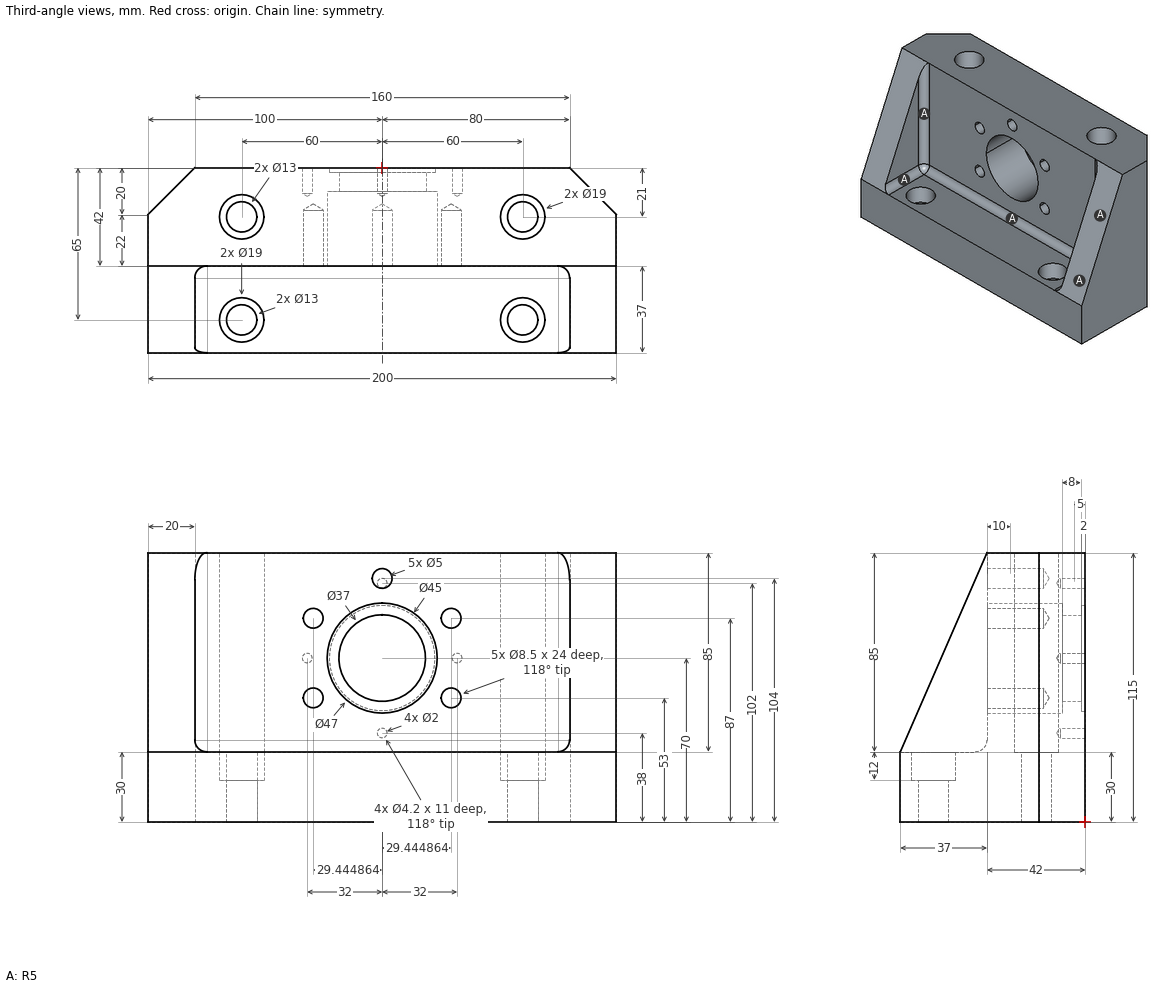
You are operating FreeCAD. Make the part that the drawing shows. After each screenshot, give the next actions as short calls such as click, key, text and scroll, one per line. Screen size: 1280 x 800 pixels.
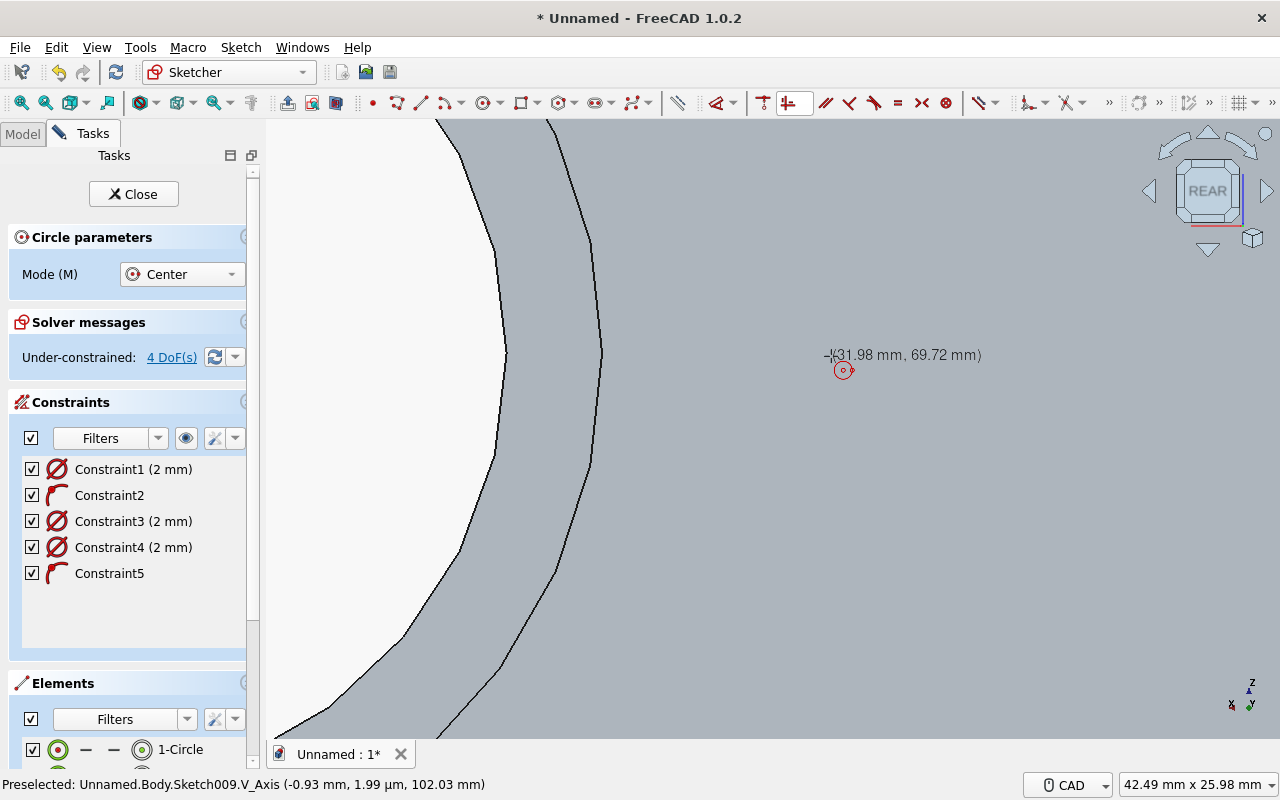
scroll(831, 357, down, 9)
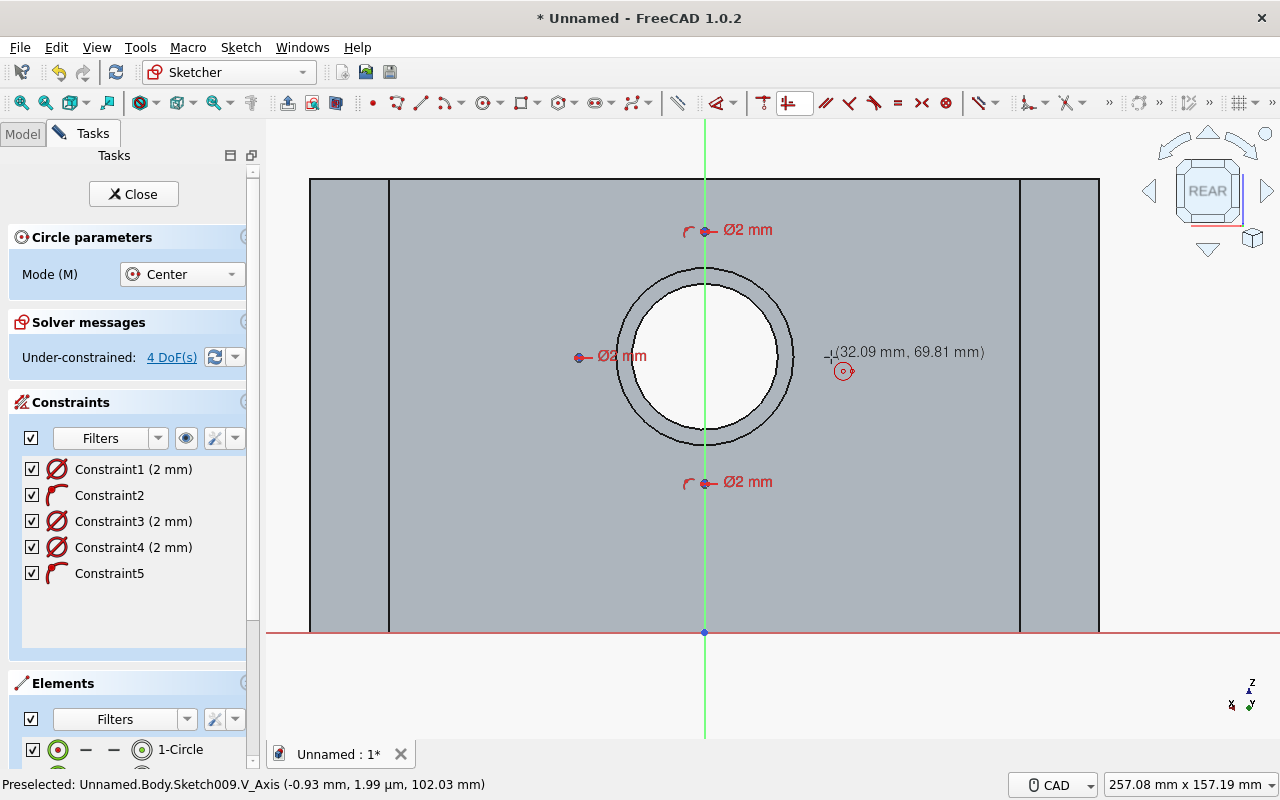
click(831, 357)
move(834, 354)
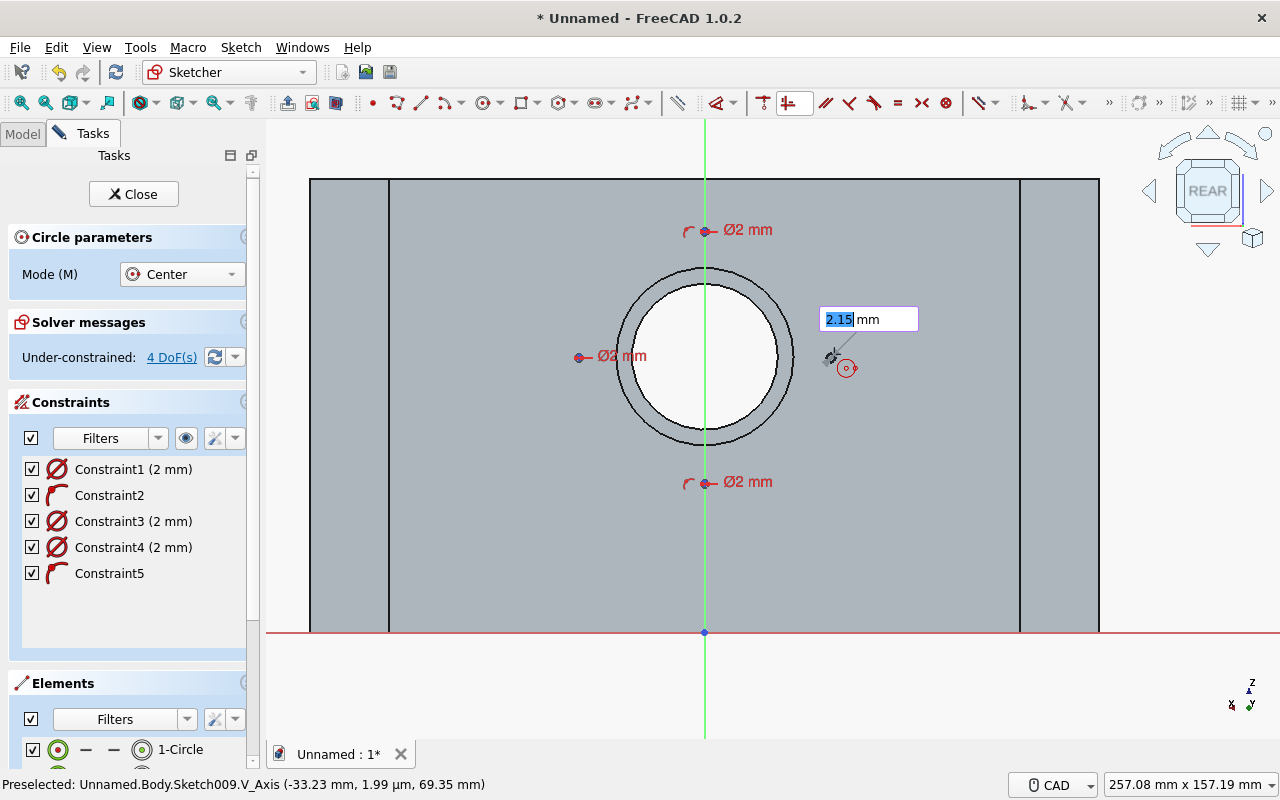
text(2)
key(Return)
key(Escape)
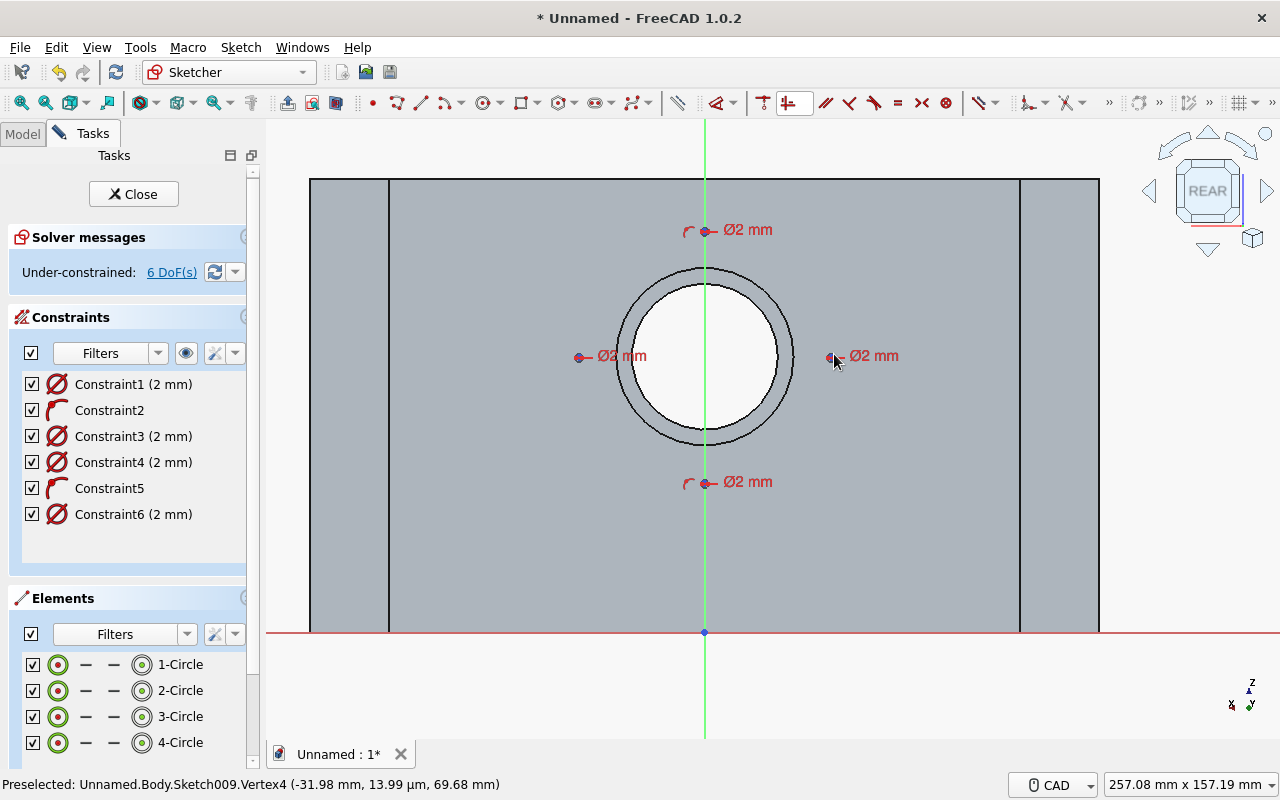
click(579, 358)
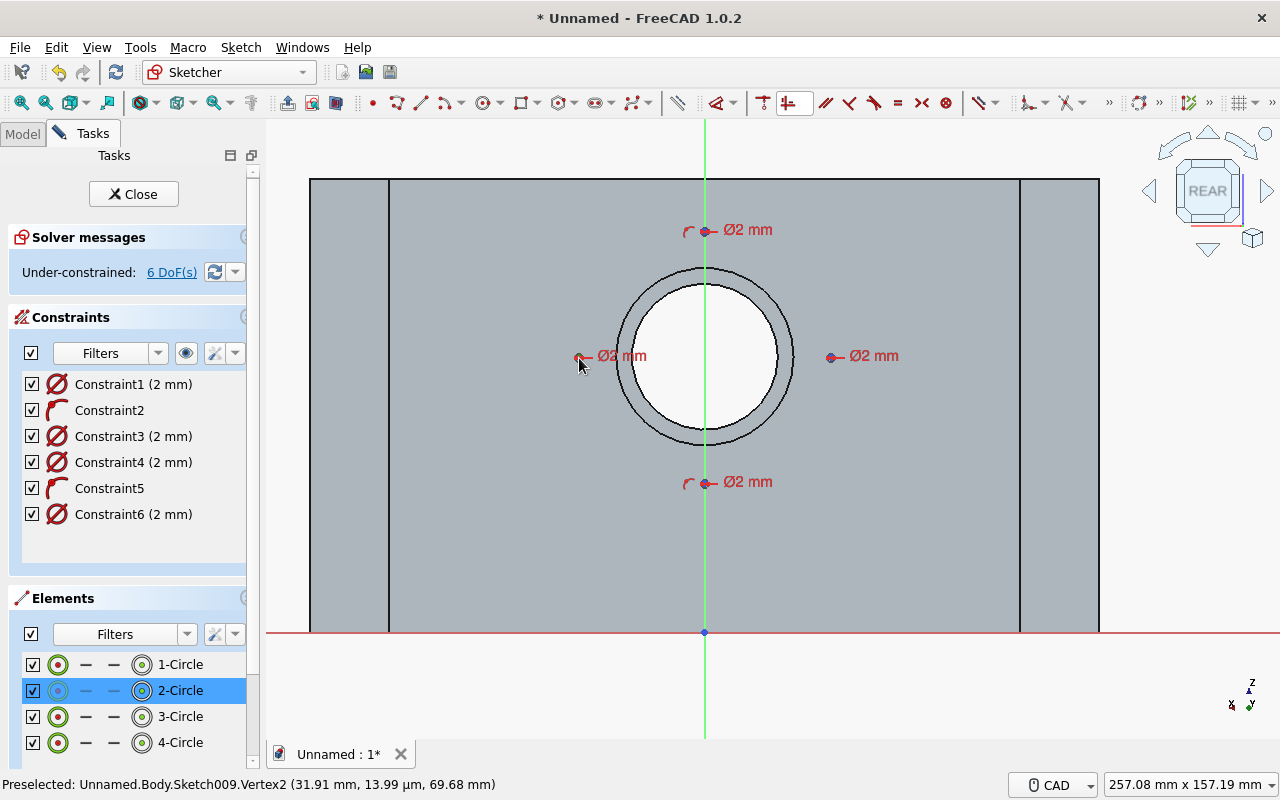
click(831, 358)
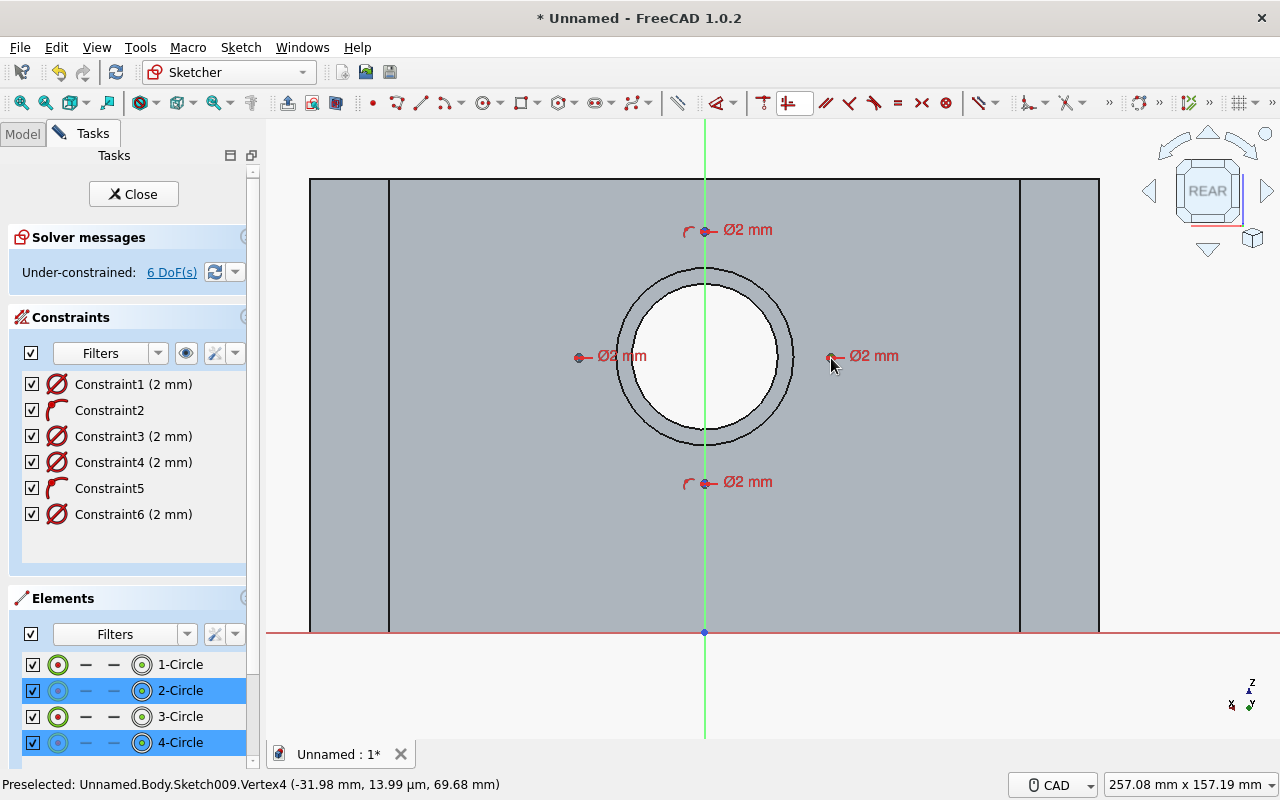
click(808, 104)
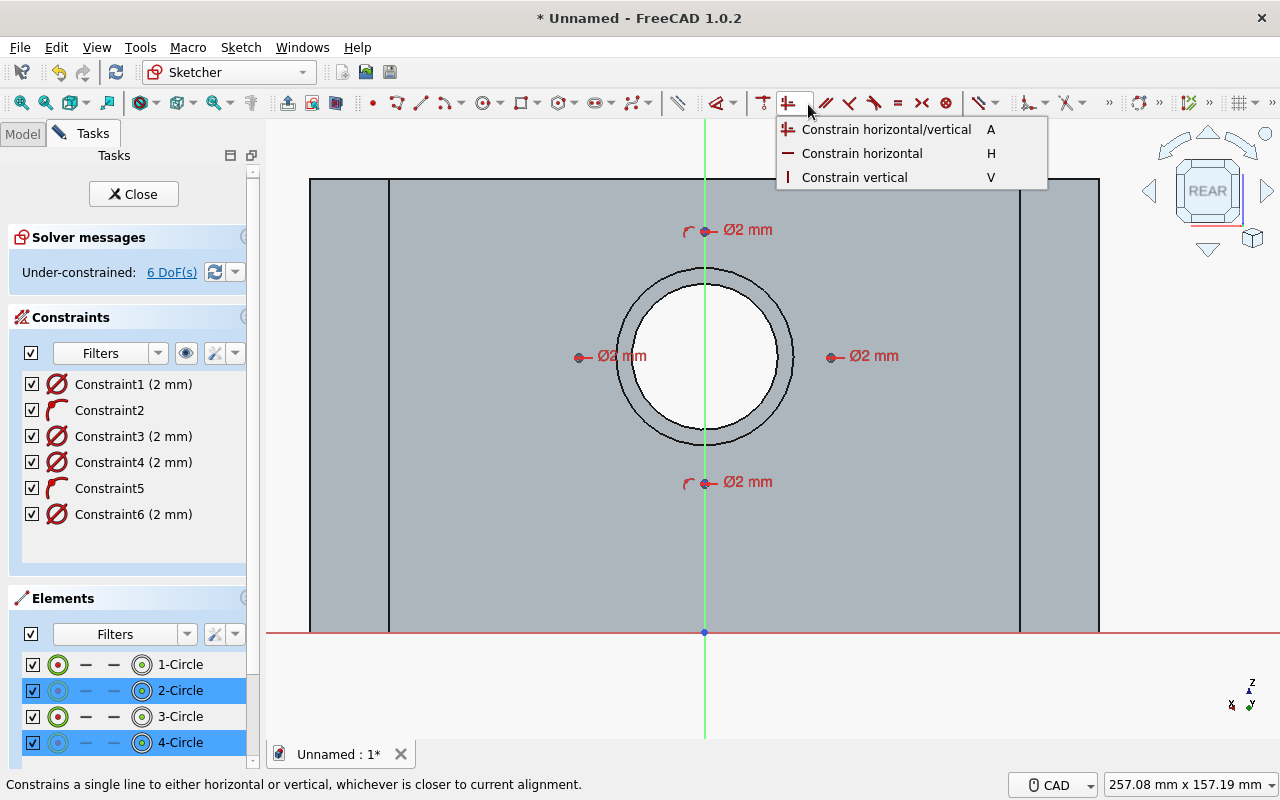
click(912, 153)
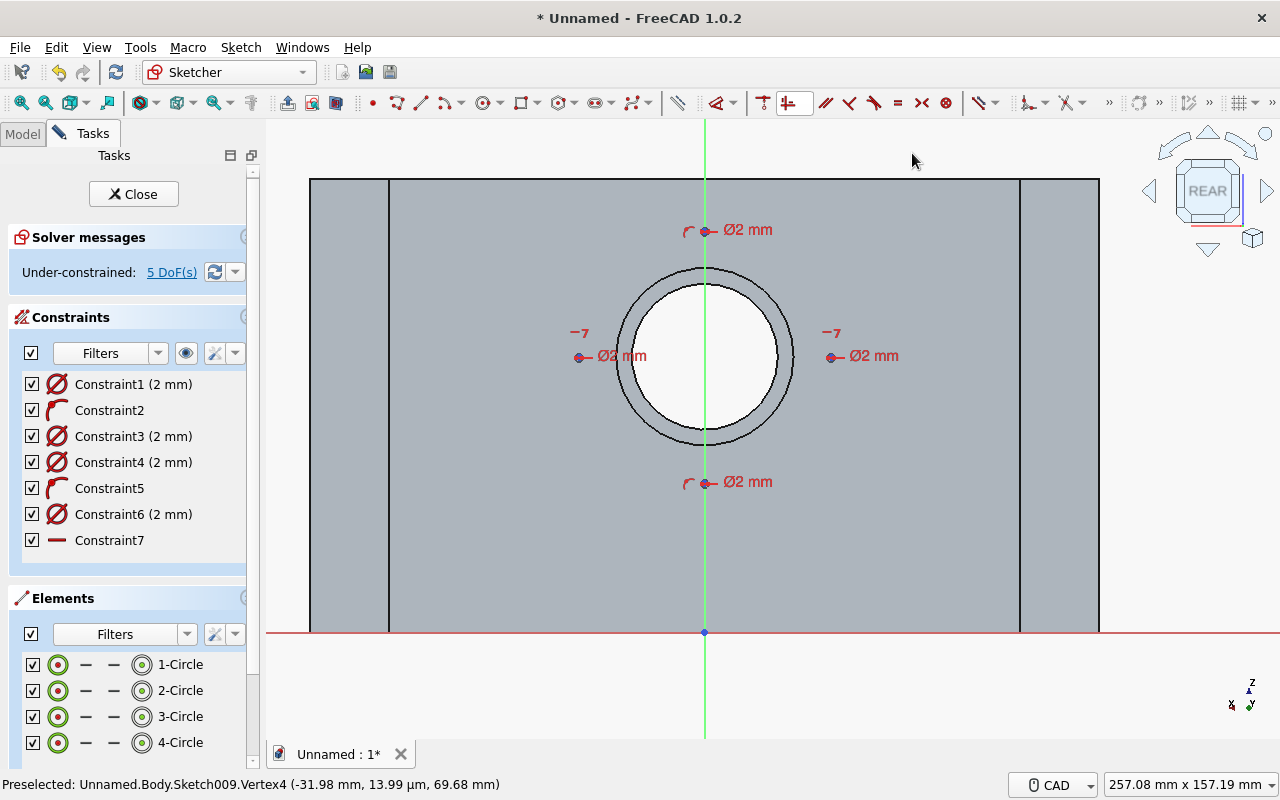
key(d)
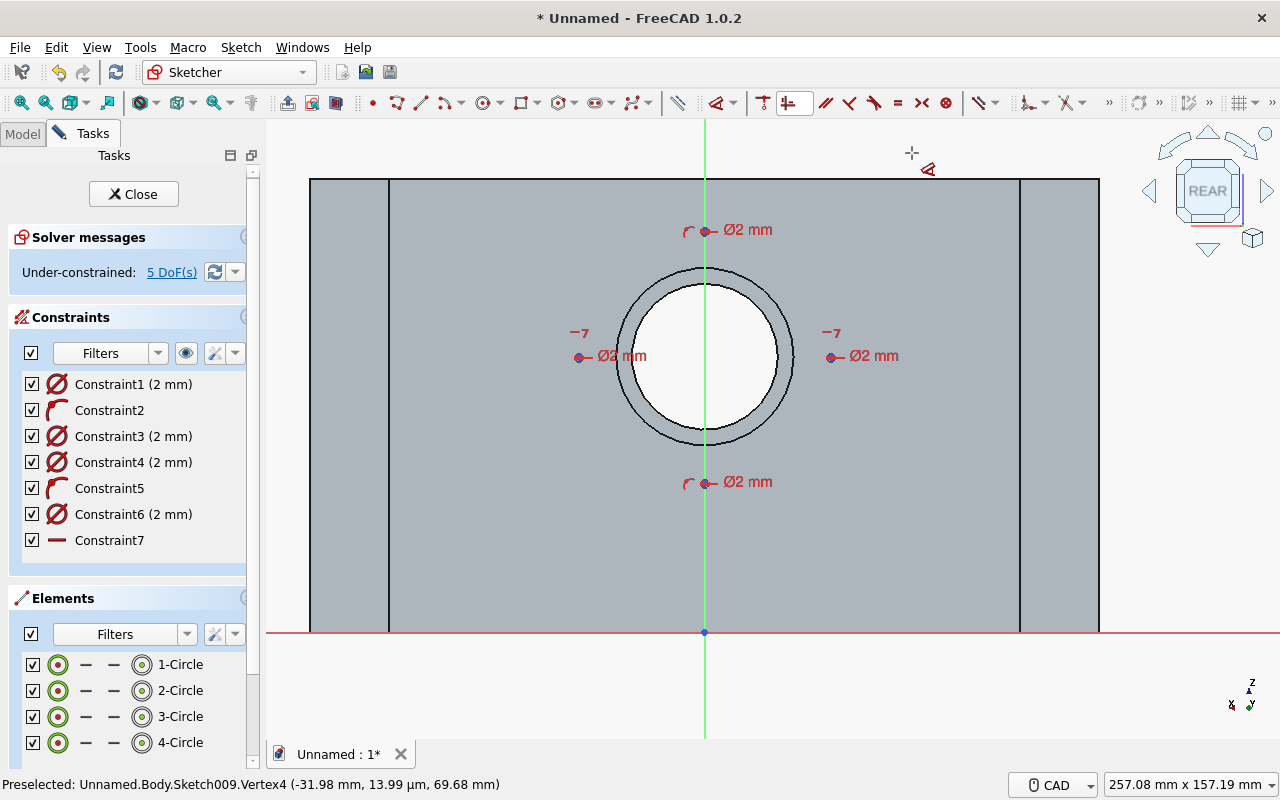
click(705, 484)
click(739, 558)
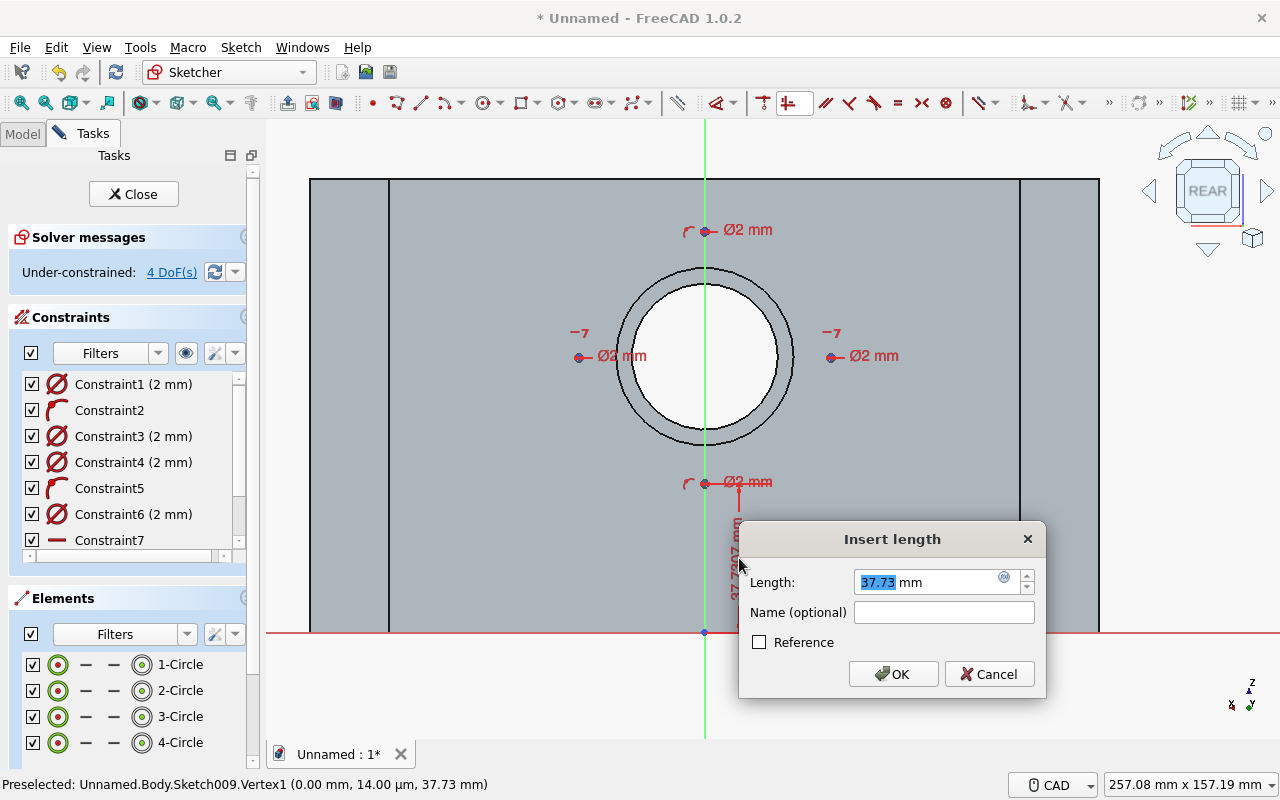
text(38)
key(Return)